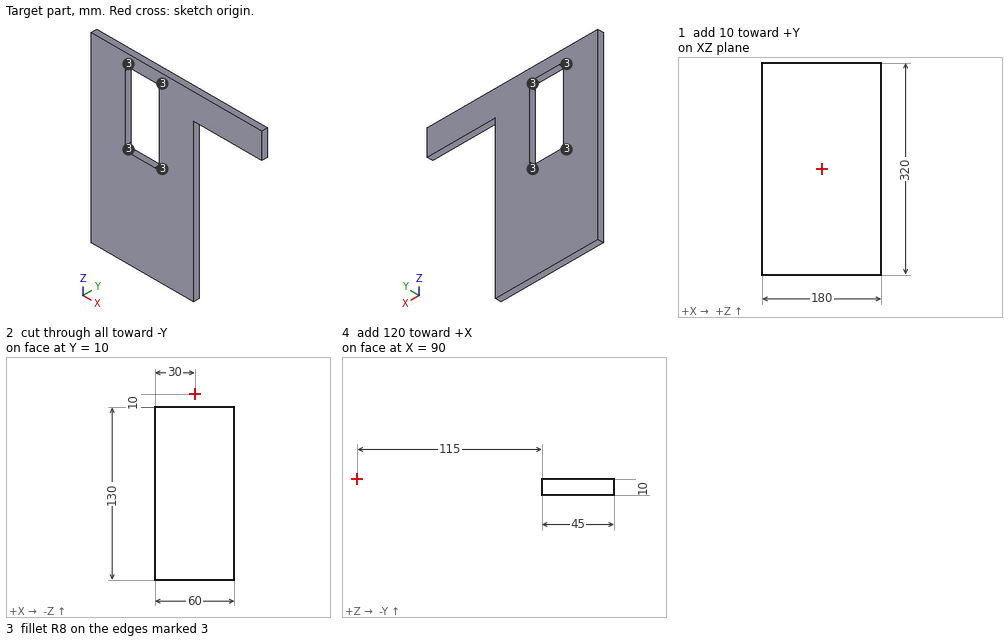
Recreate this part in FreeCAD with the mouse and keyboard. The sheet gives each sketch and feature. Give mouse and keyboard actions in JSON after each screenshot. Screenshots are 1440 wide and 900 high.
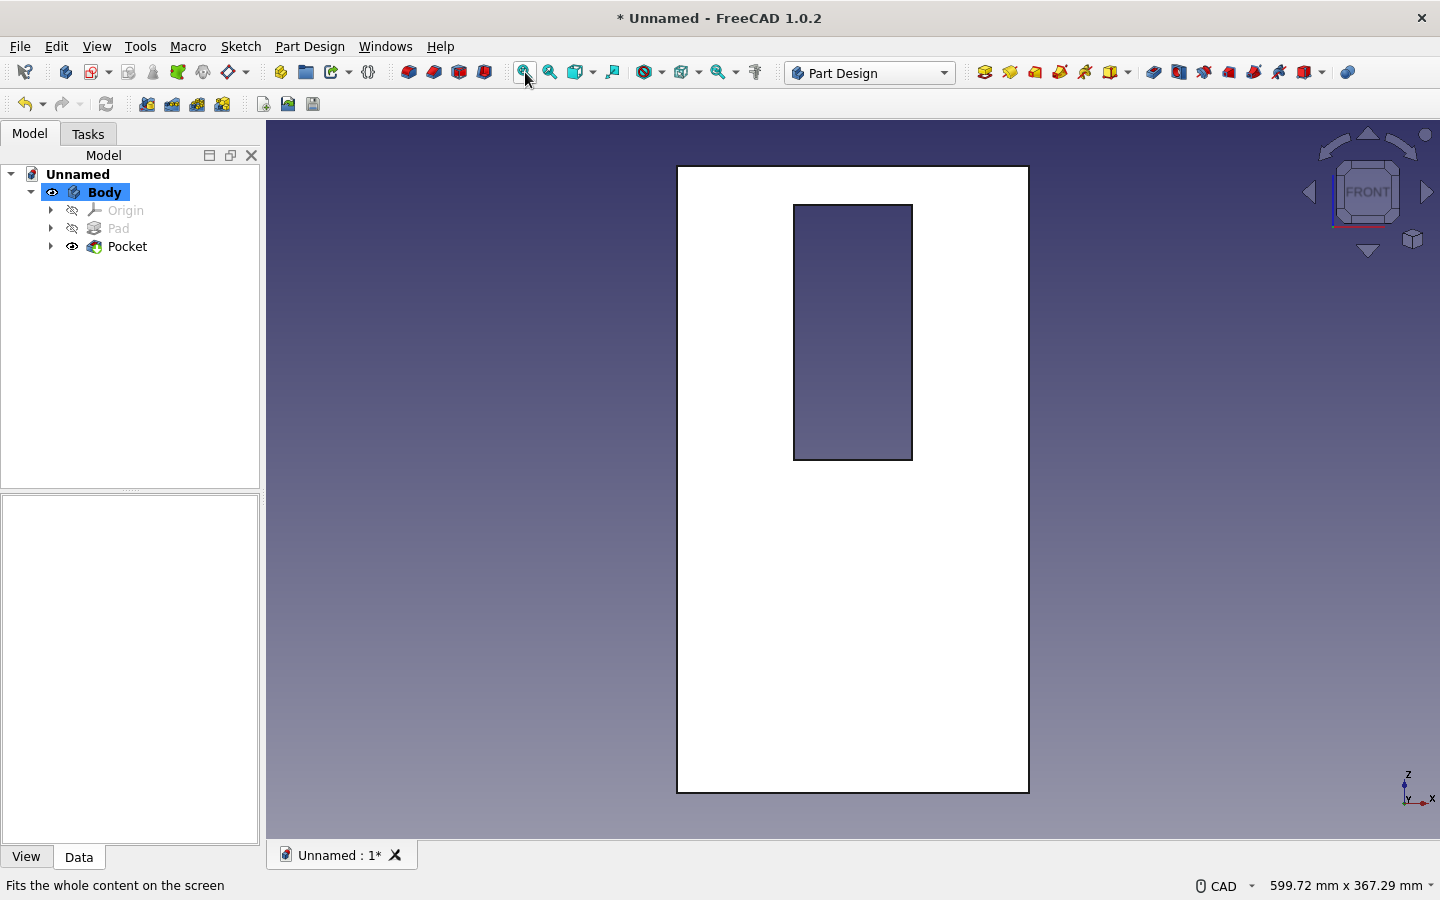
{"action": "scroll", "coordinate": [912, 459], "scroll_direction": "up", "scroll_amount": 4}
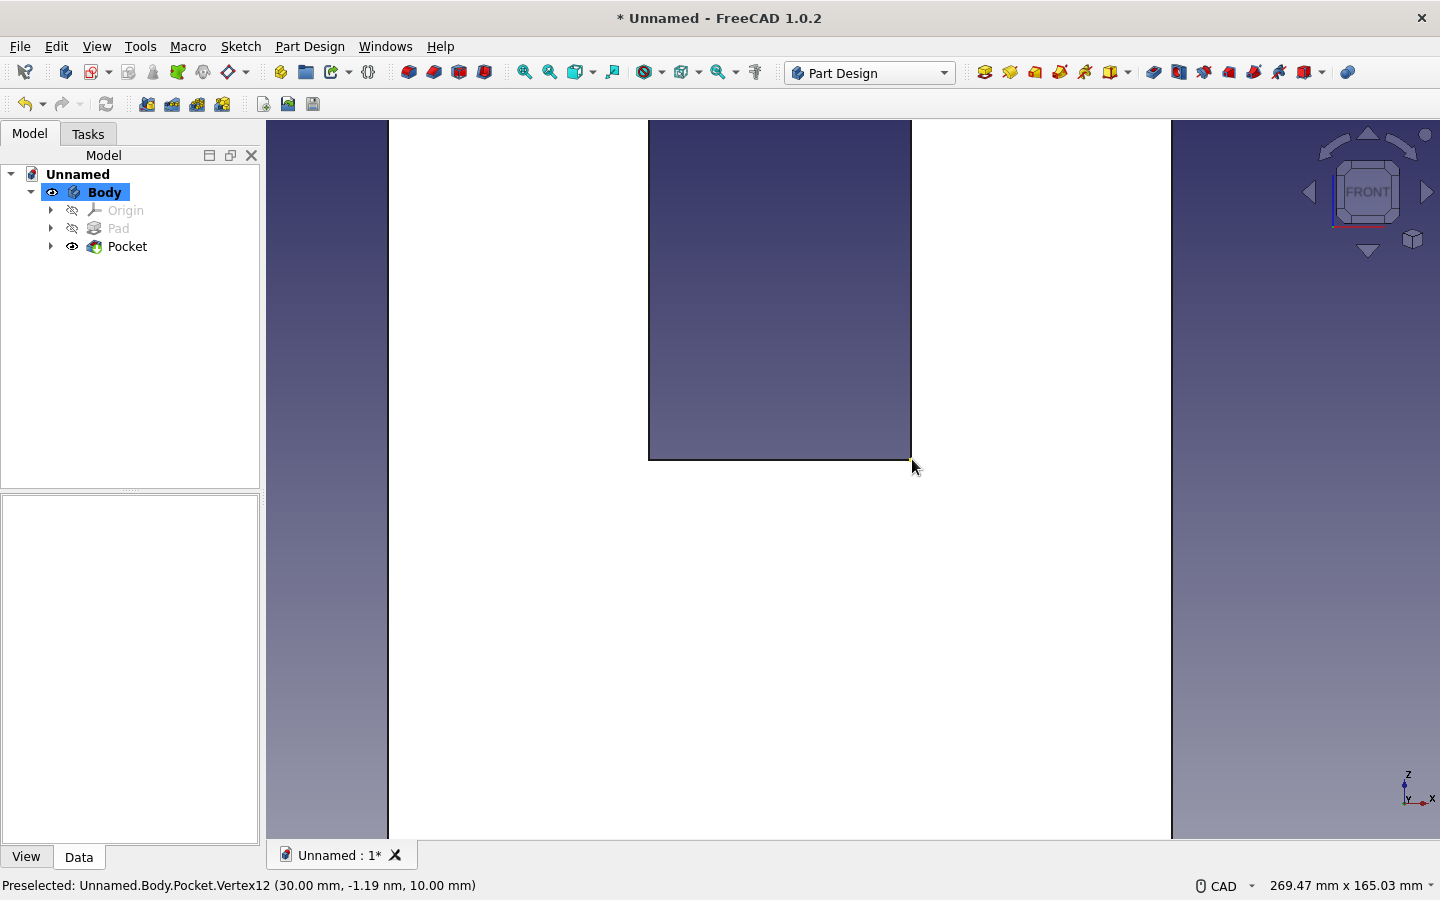
{"action": "left_click", "coordinate": [525, 72]}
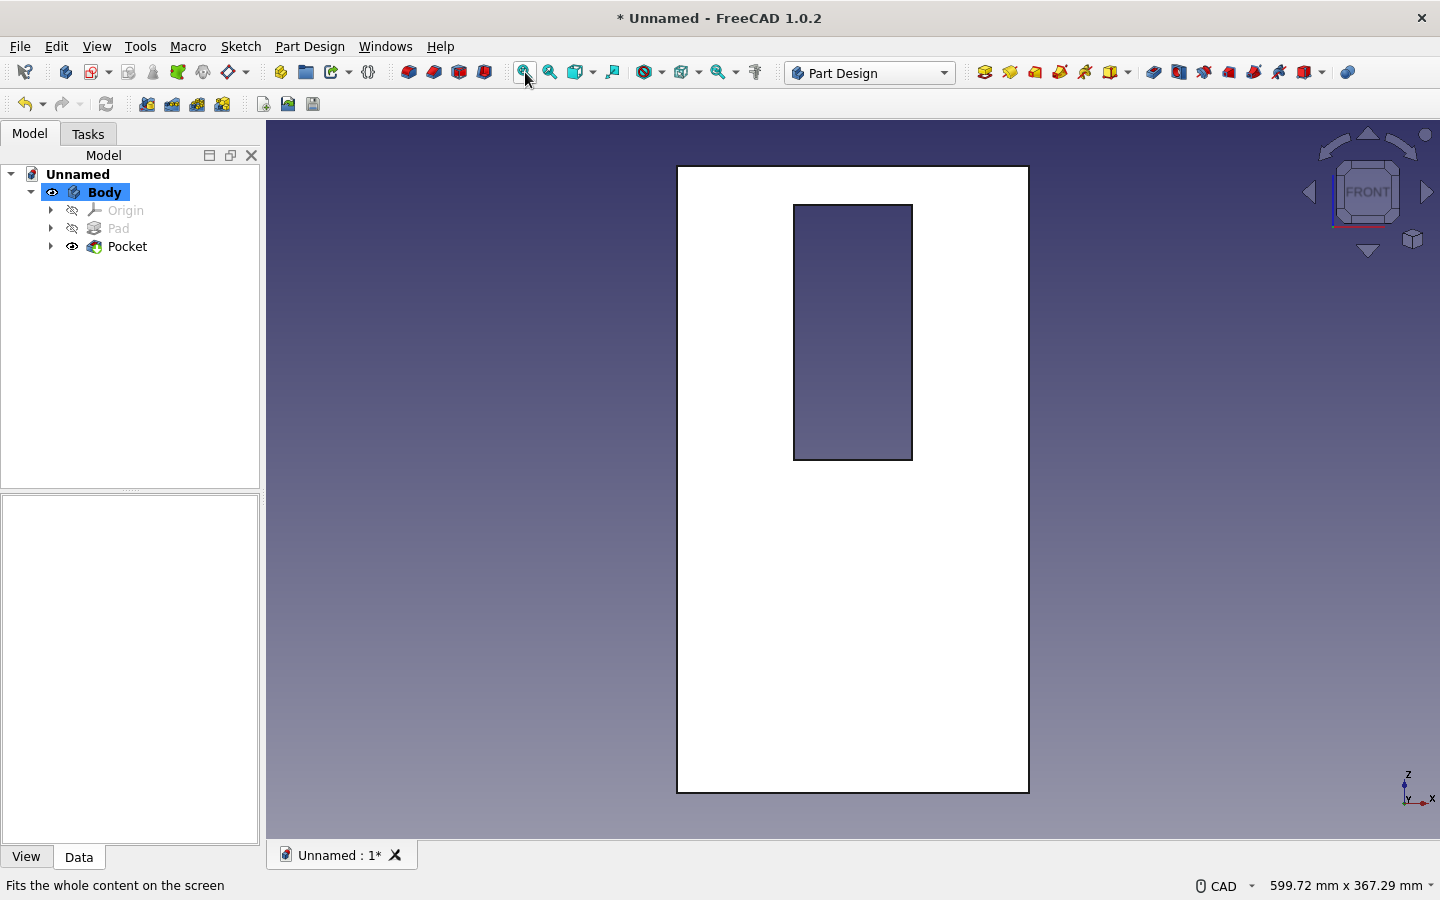
{"action": "key", "text": "3"}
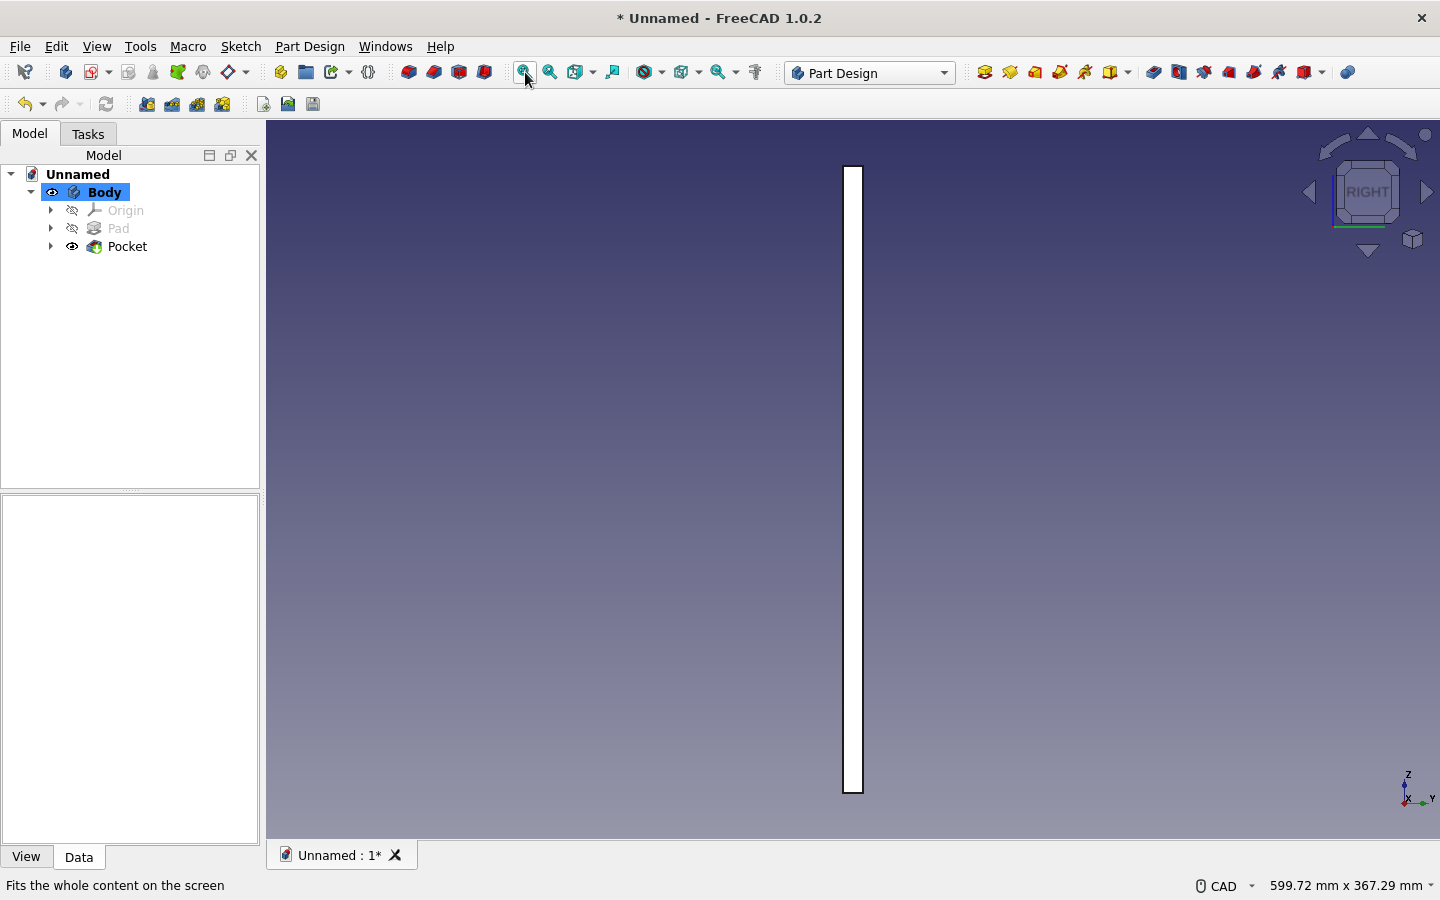
{"action": "scroll", "coordinate": [853, 459], "scroll_direction": "up", "scroll_amount": 4}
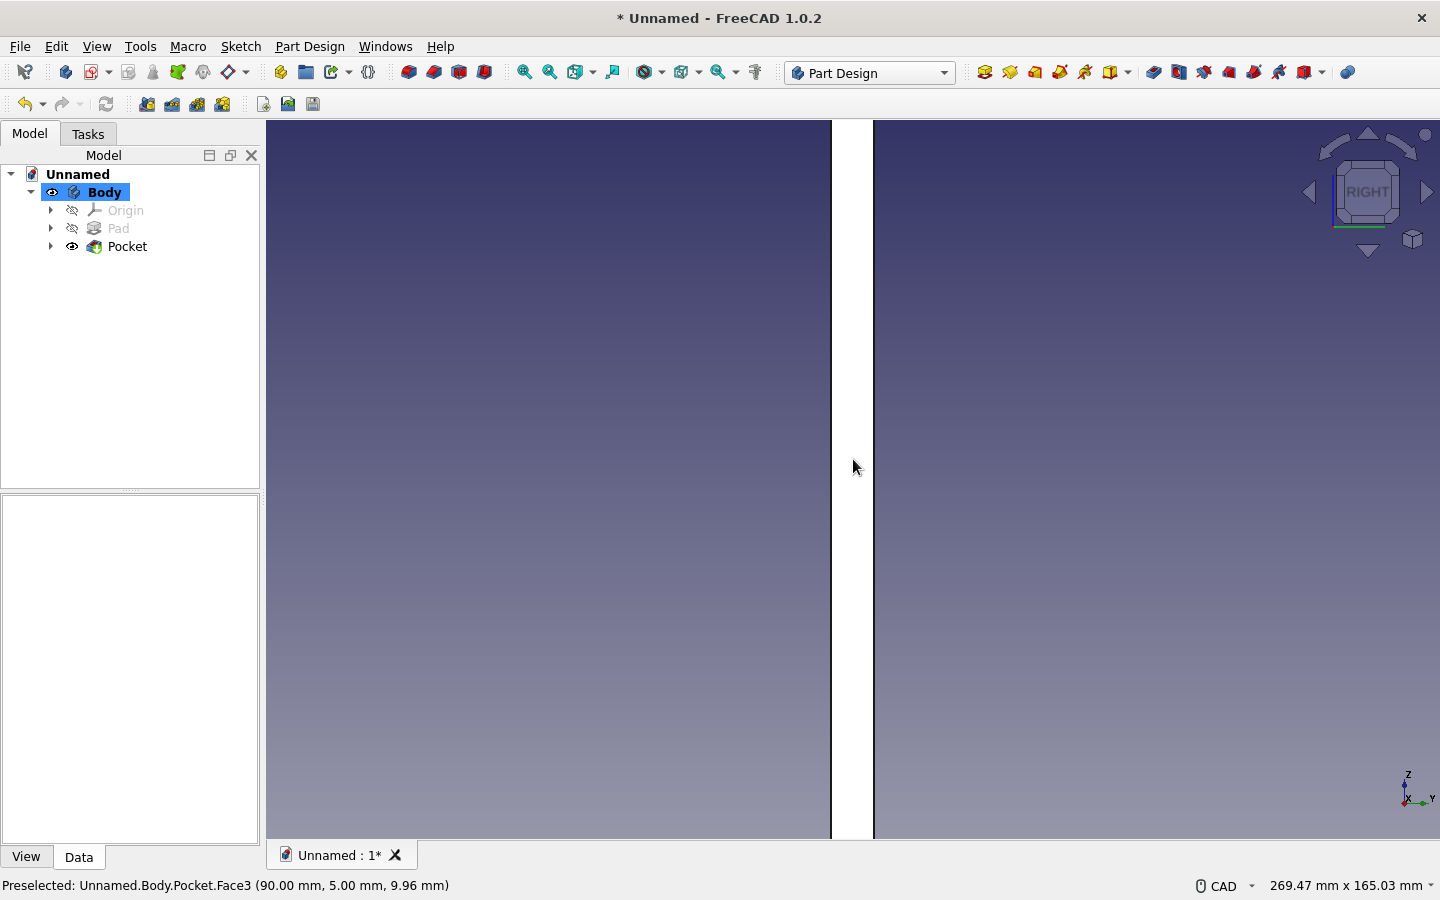
{"action": "left_click", "coordinate": [525, 72]}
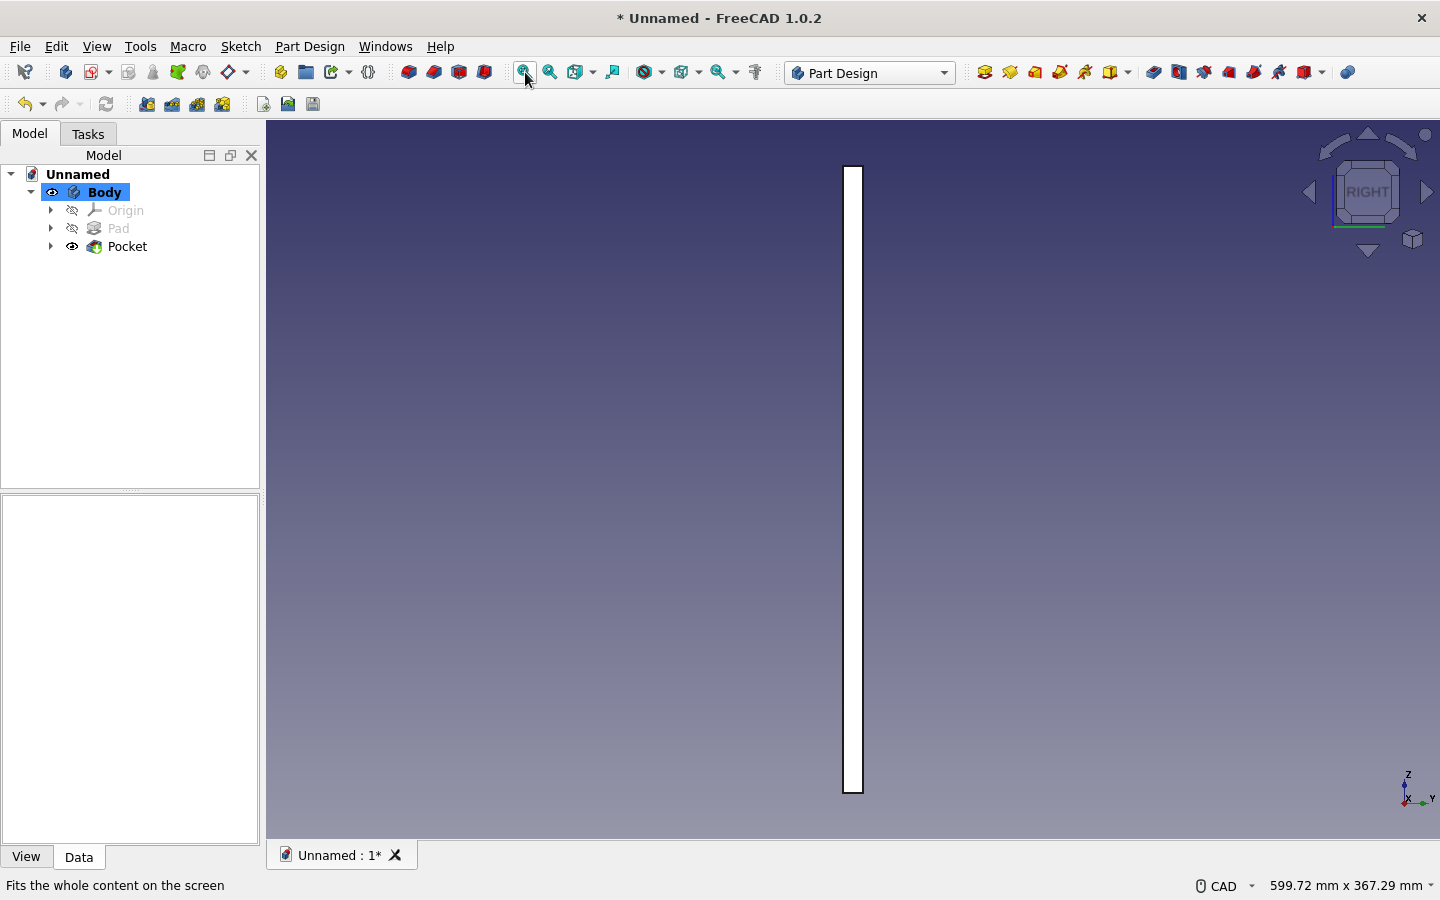
{"action": "key", "text": "5"}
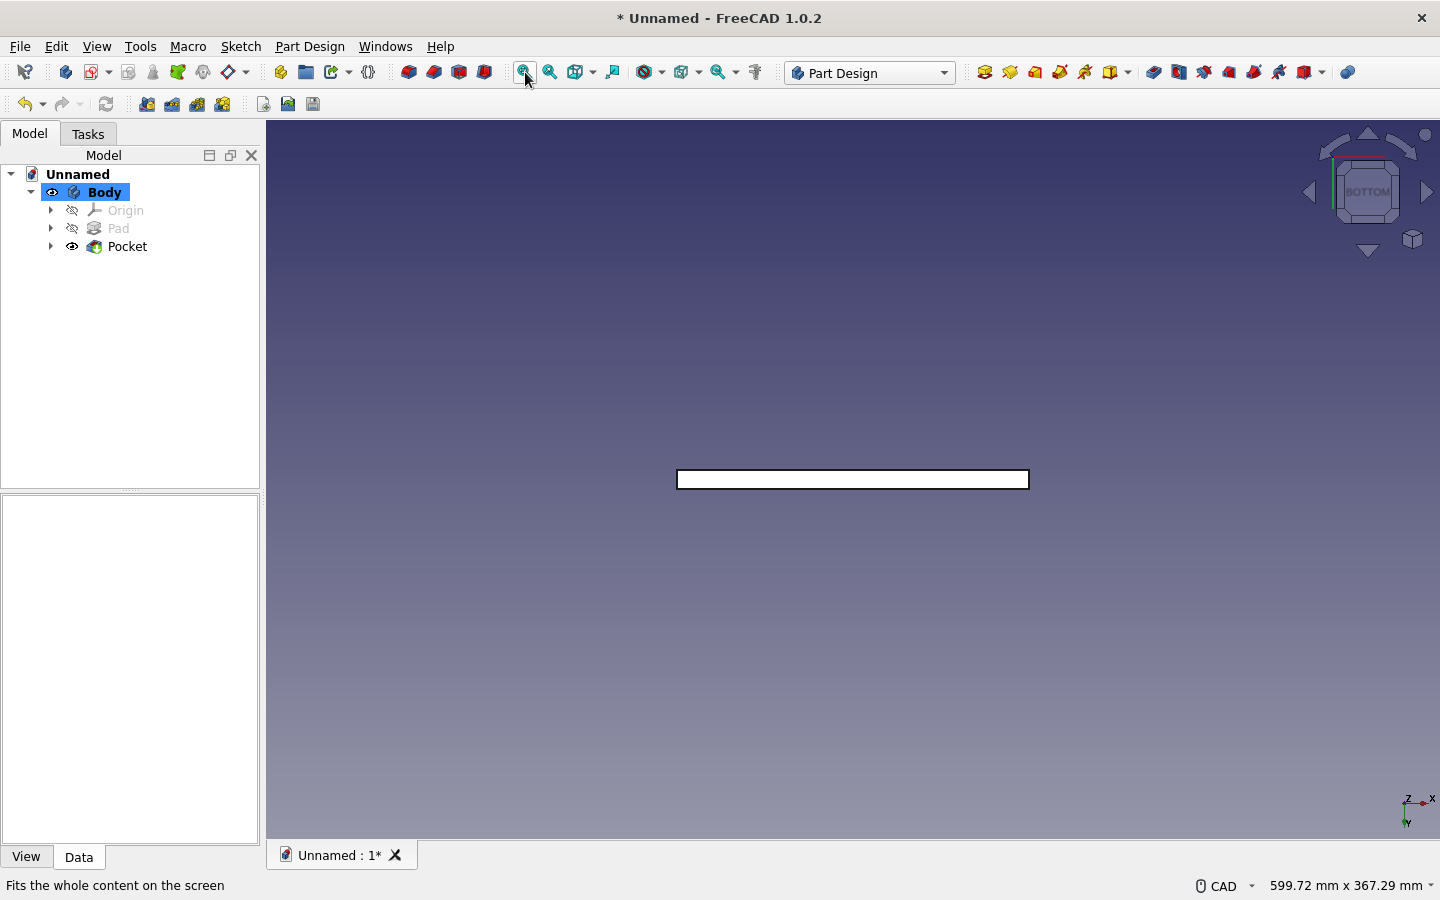
{"action": "left_click", "coordinate": [525, 72]}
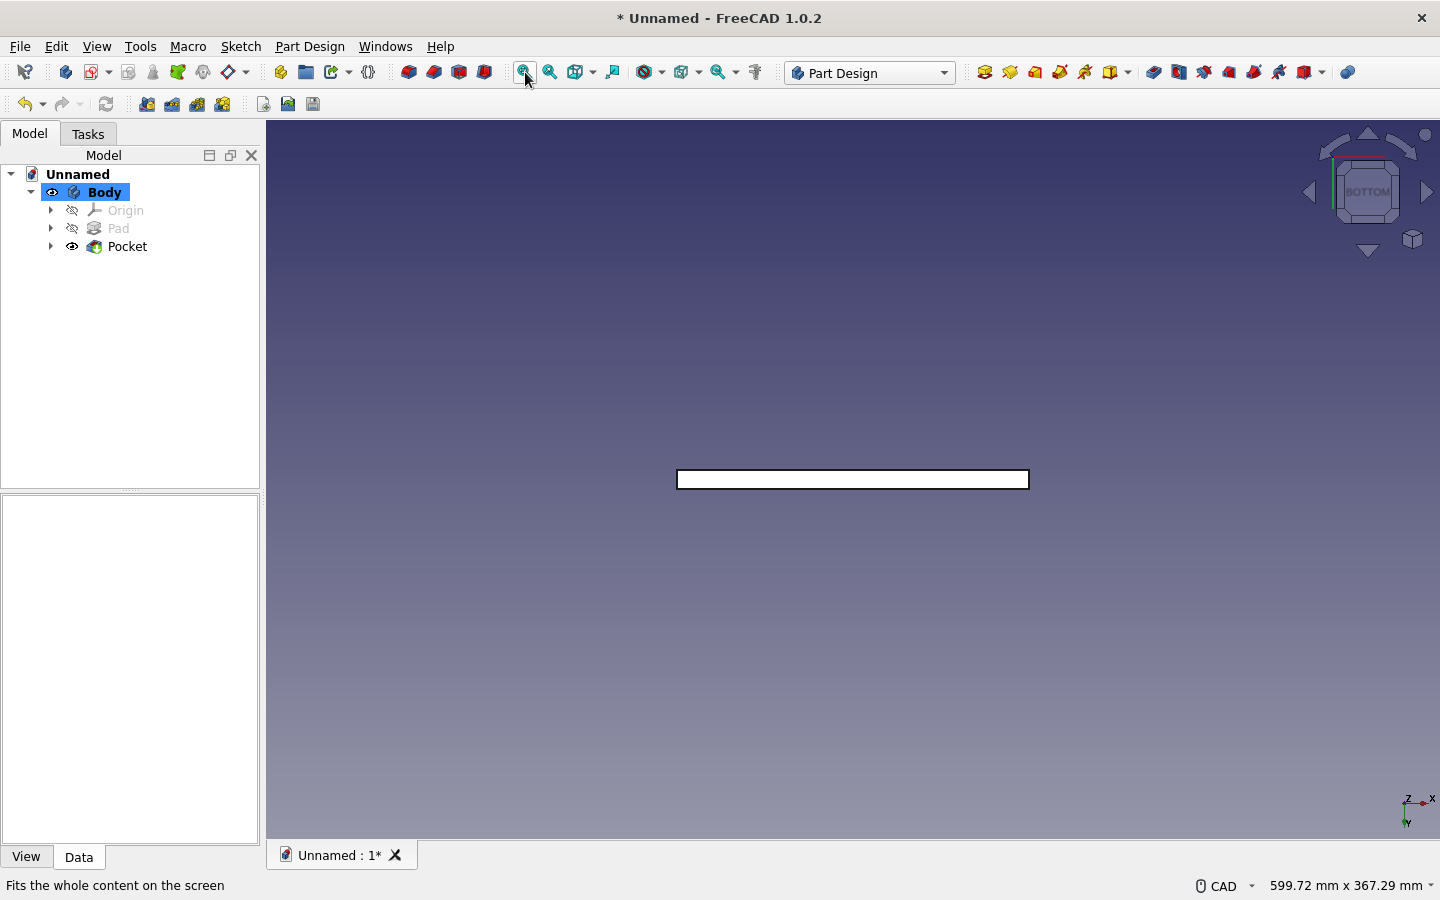
{"action": "scroll", "coordinate": [912, 478], "scroll_direction": "up", "scroll_amount": 4}